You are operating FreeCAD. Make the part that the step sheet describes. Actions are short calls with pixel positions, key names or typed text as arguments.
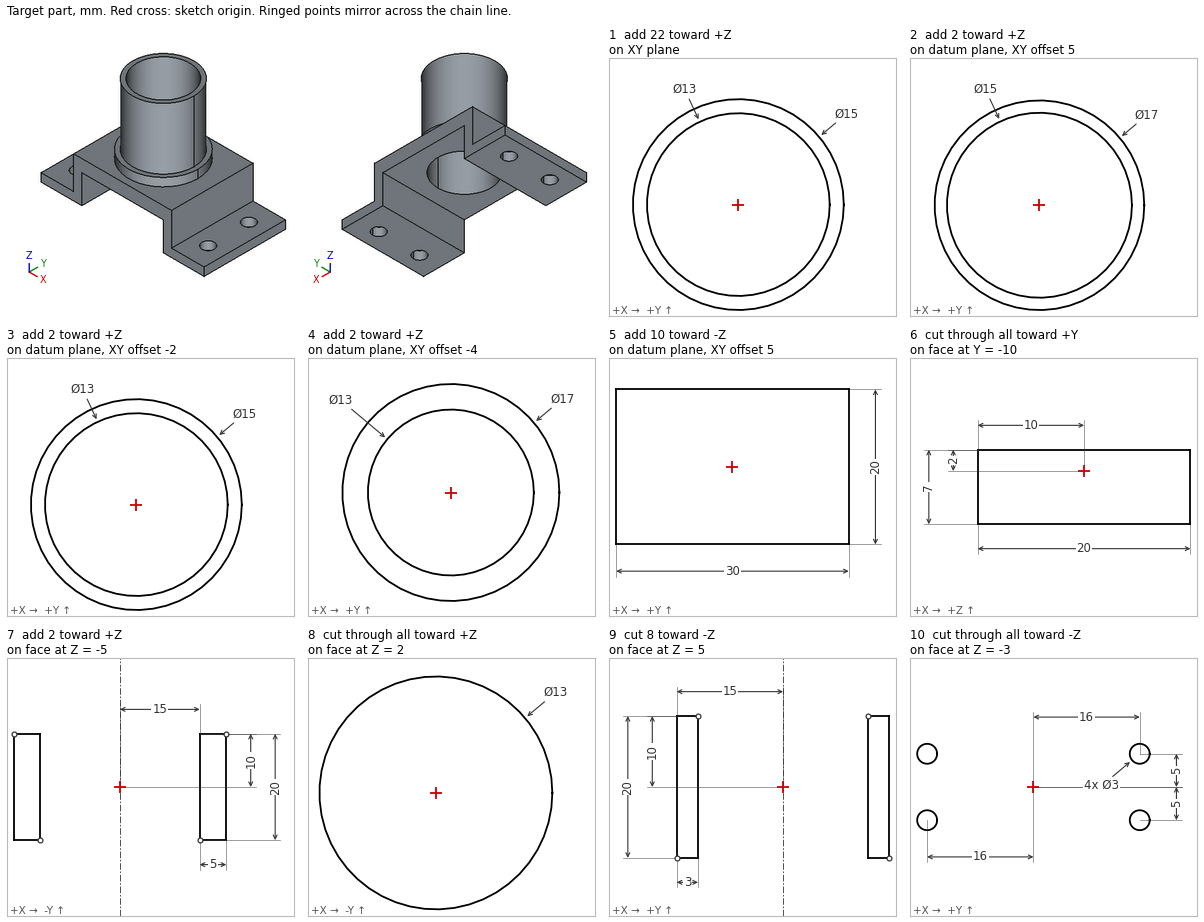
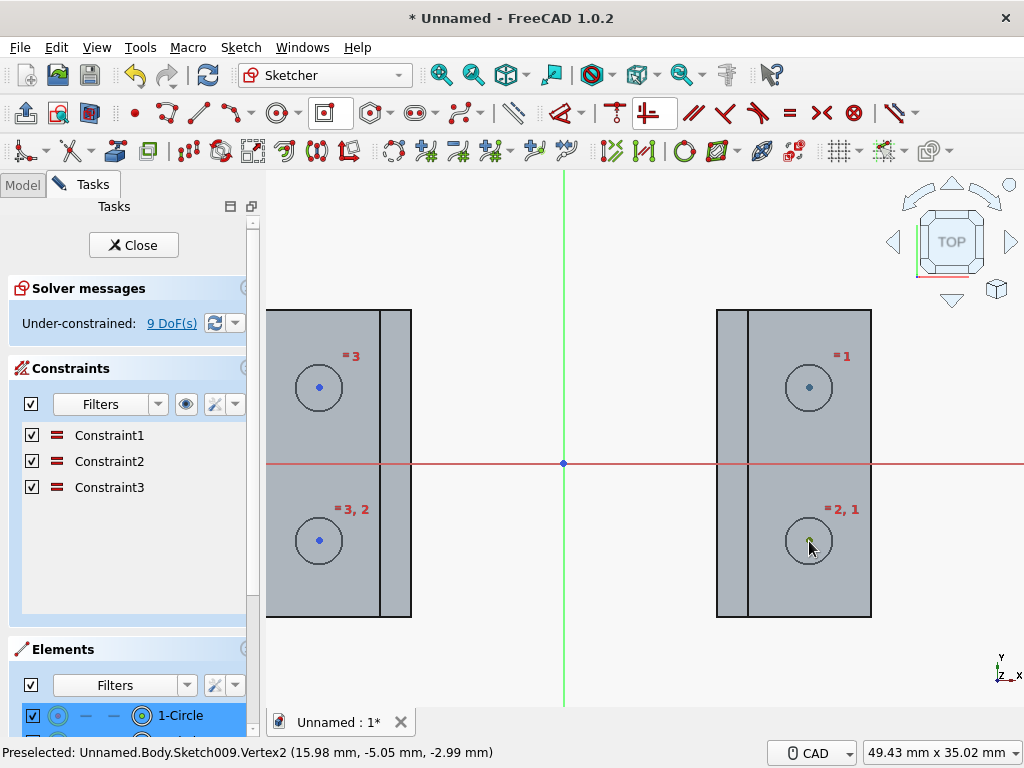
key(v)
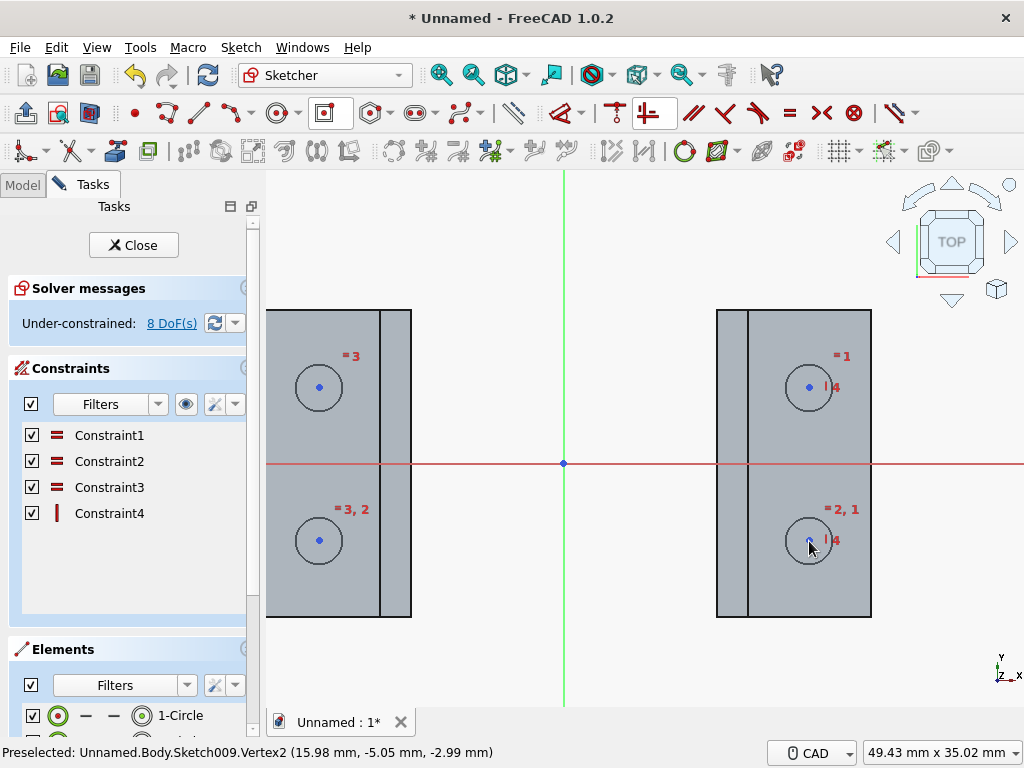
click(809, 541)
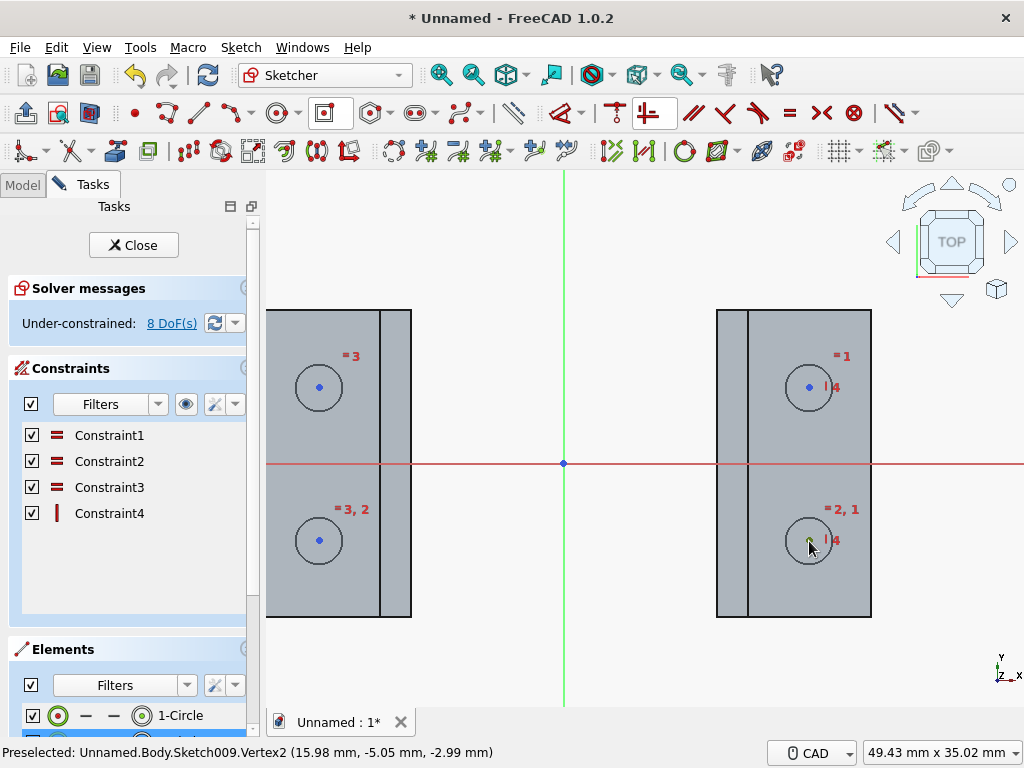
click(319, 541)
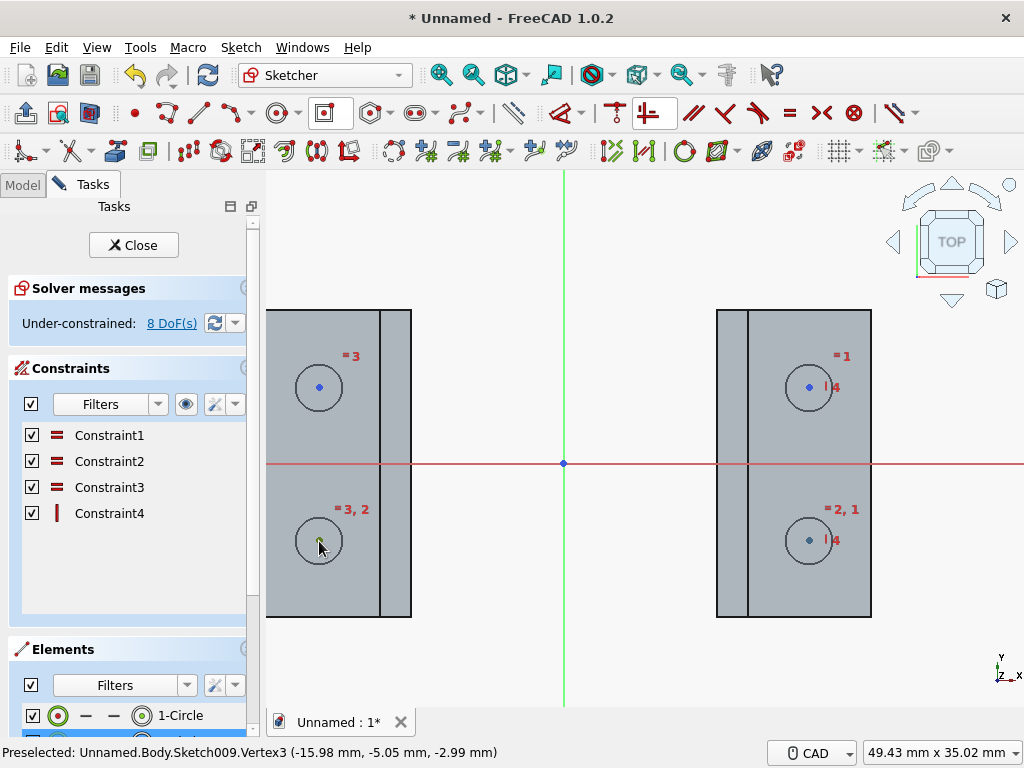
key(h)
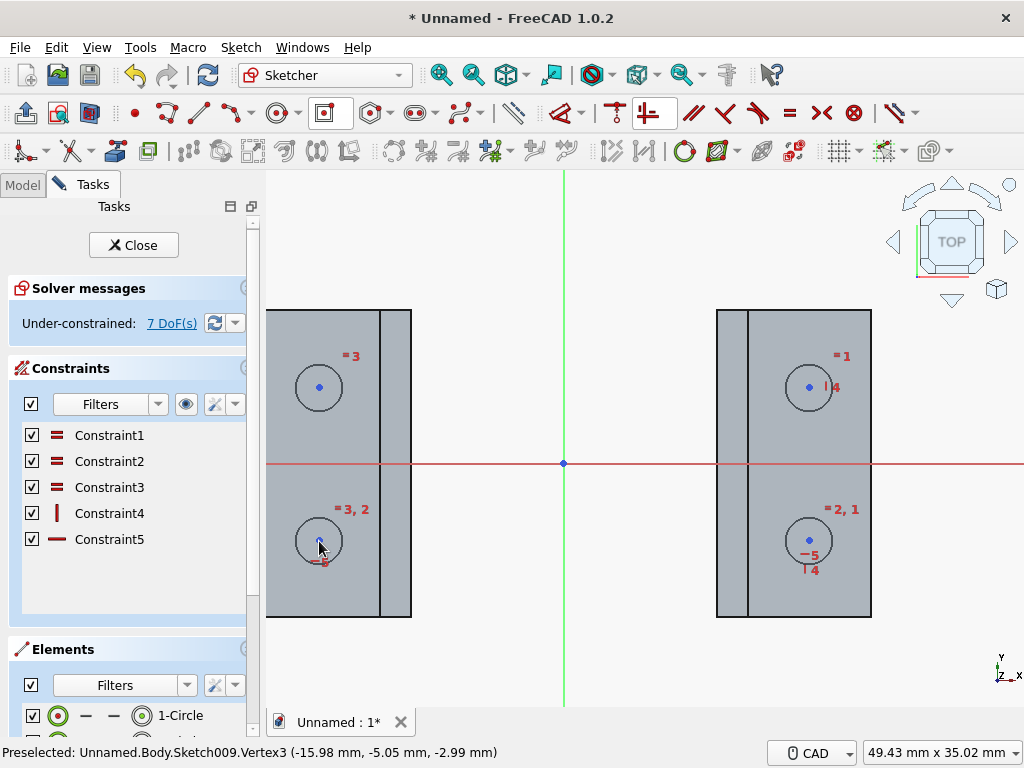
click(319, 541)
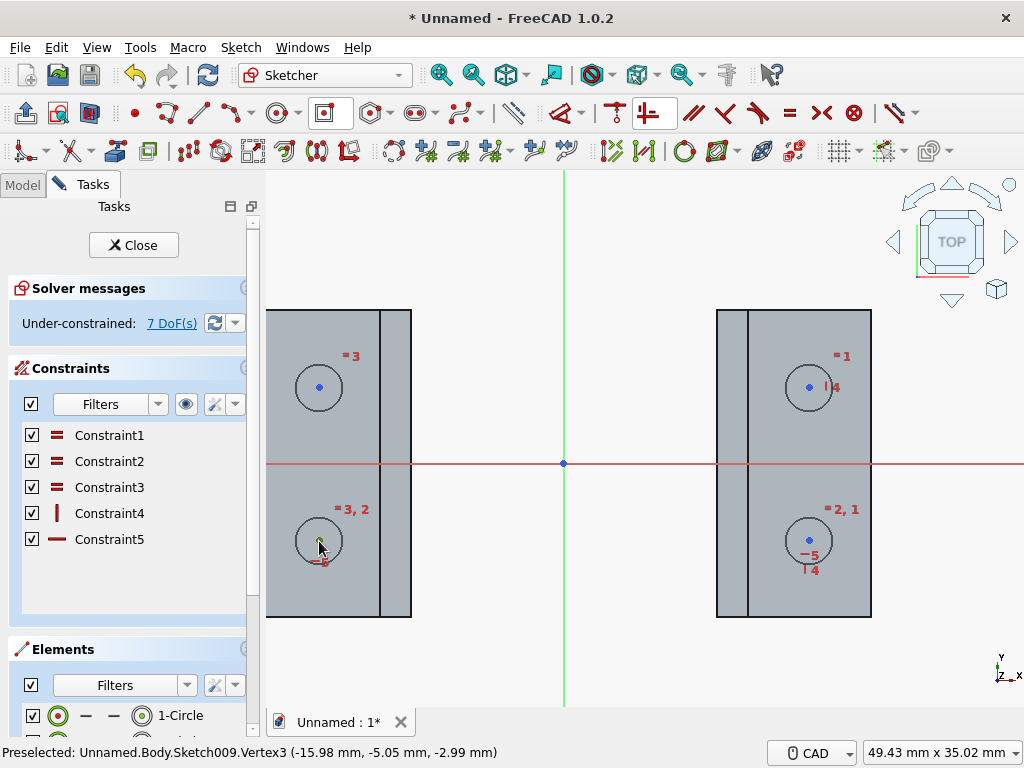
click(319, 388)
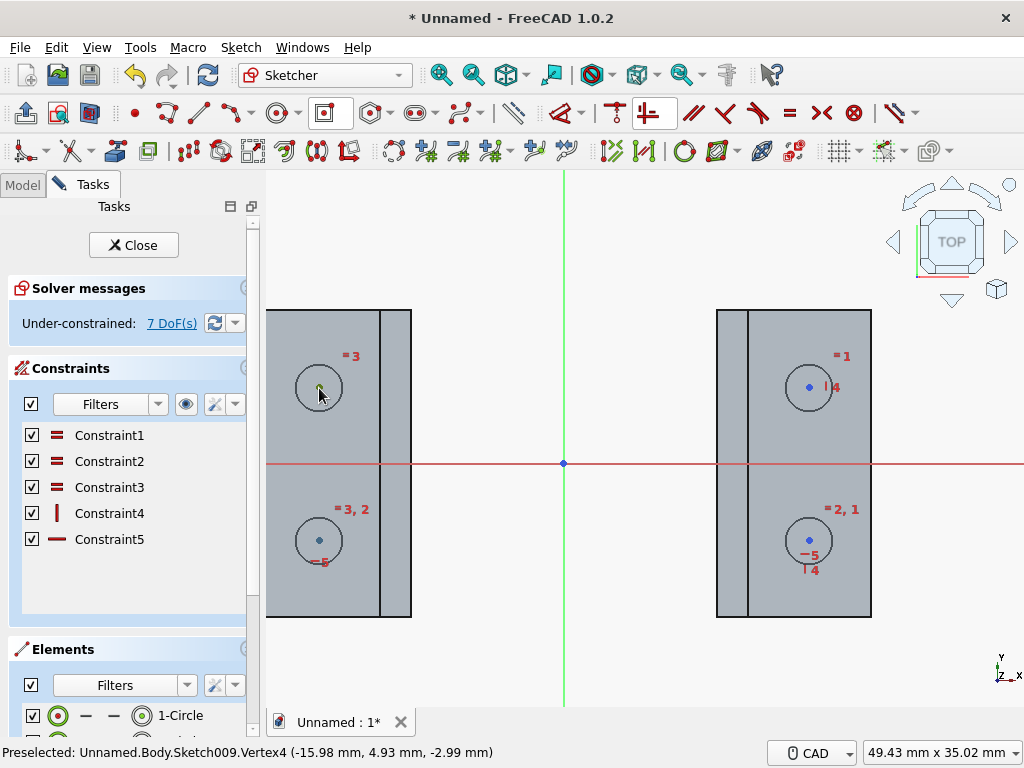
click(672, 114)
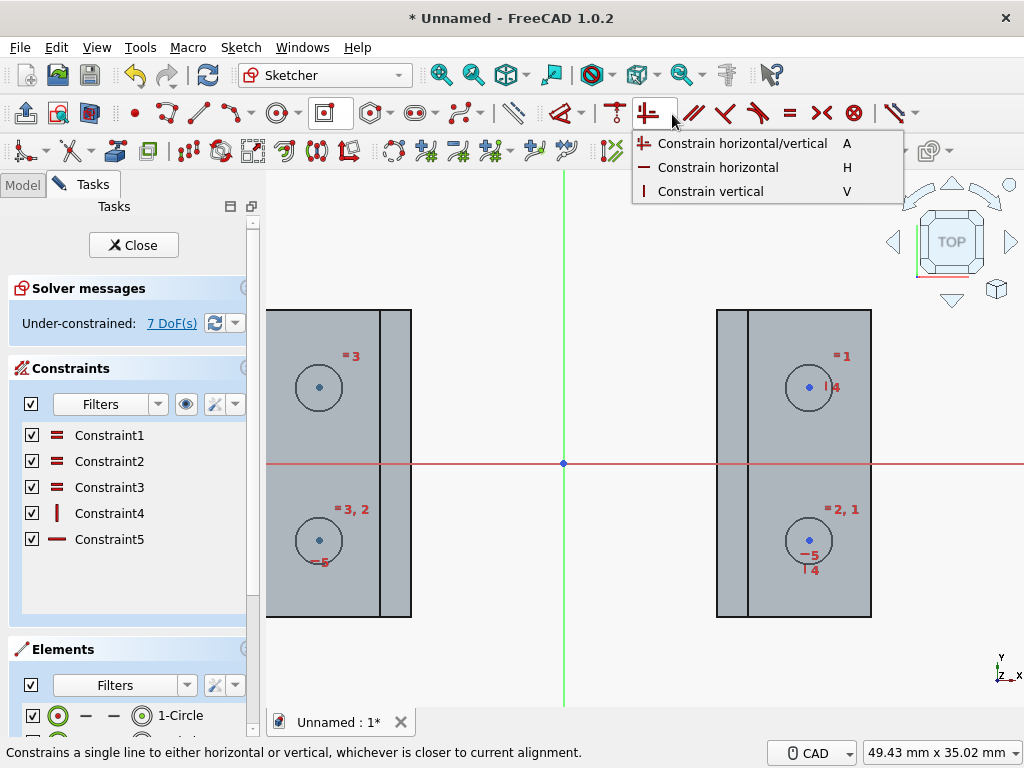
click(768, 191)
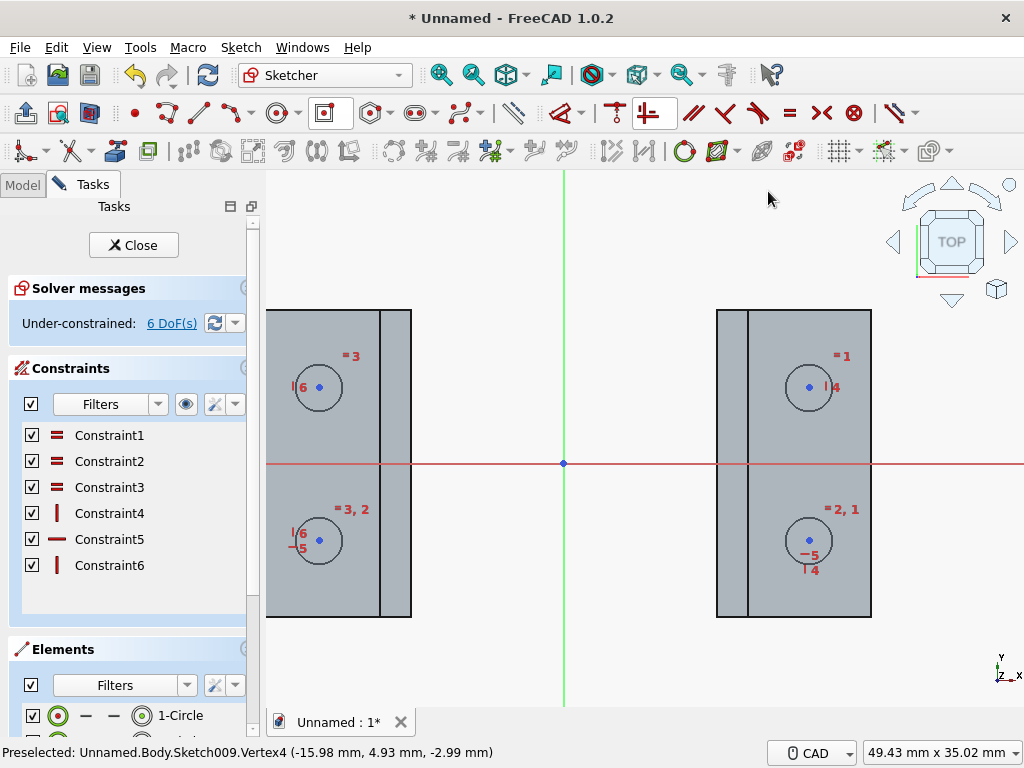
click(809, 388)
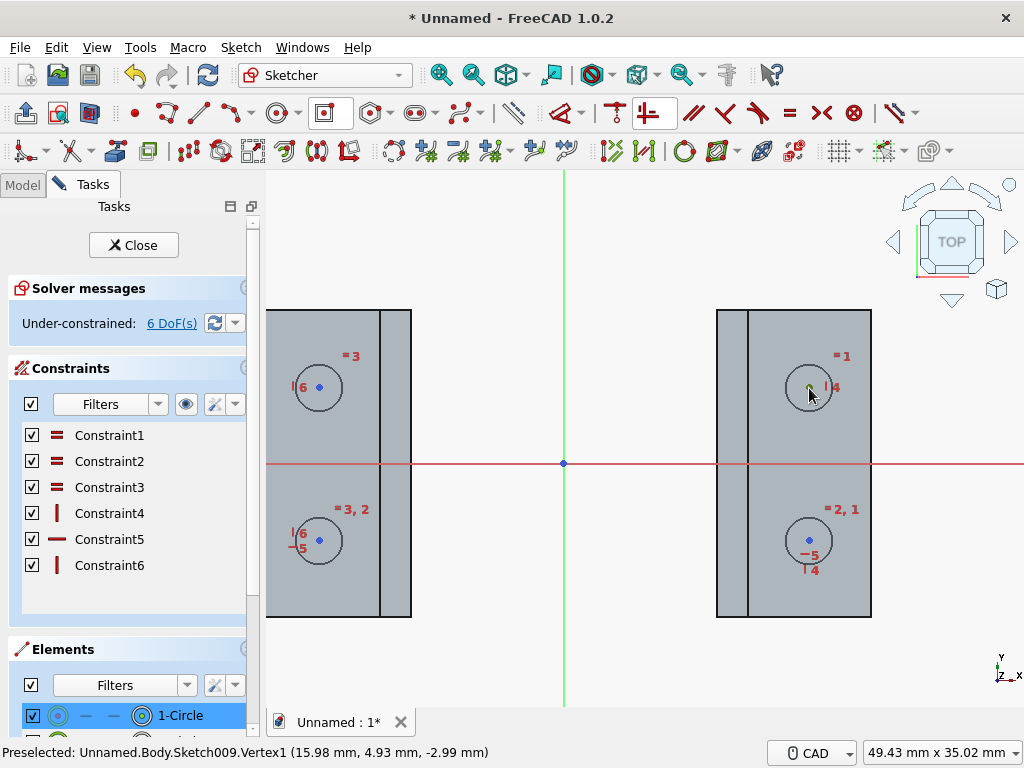
click(319, 388)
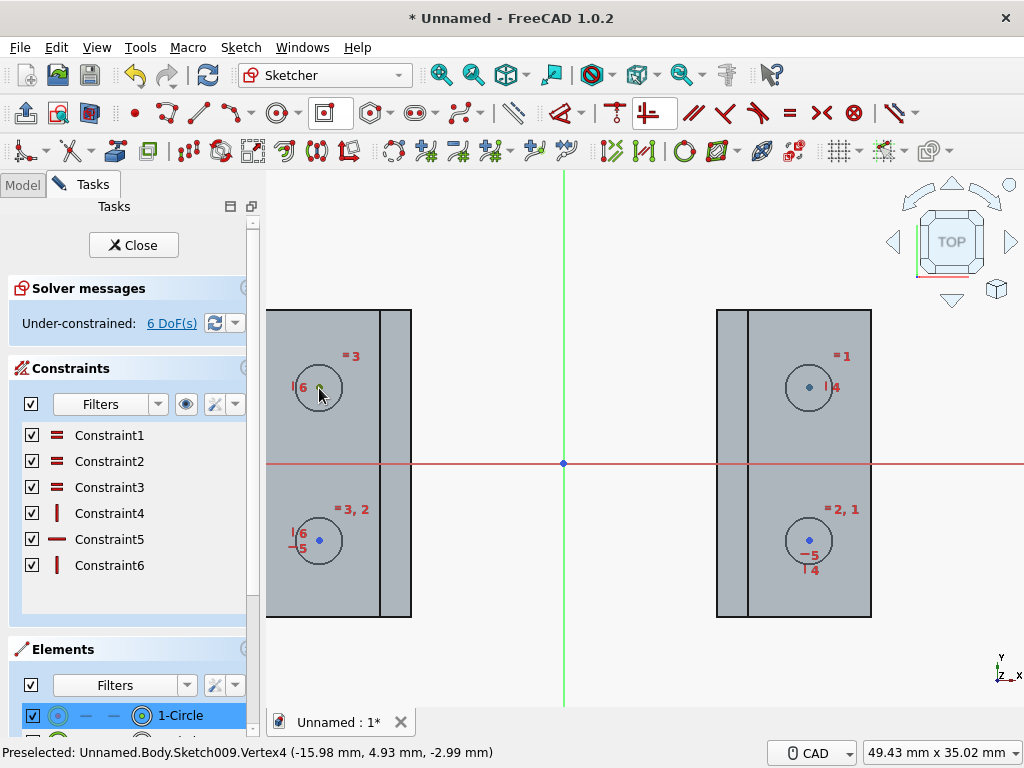
click(672, 114)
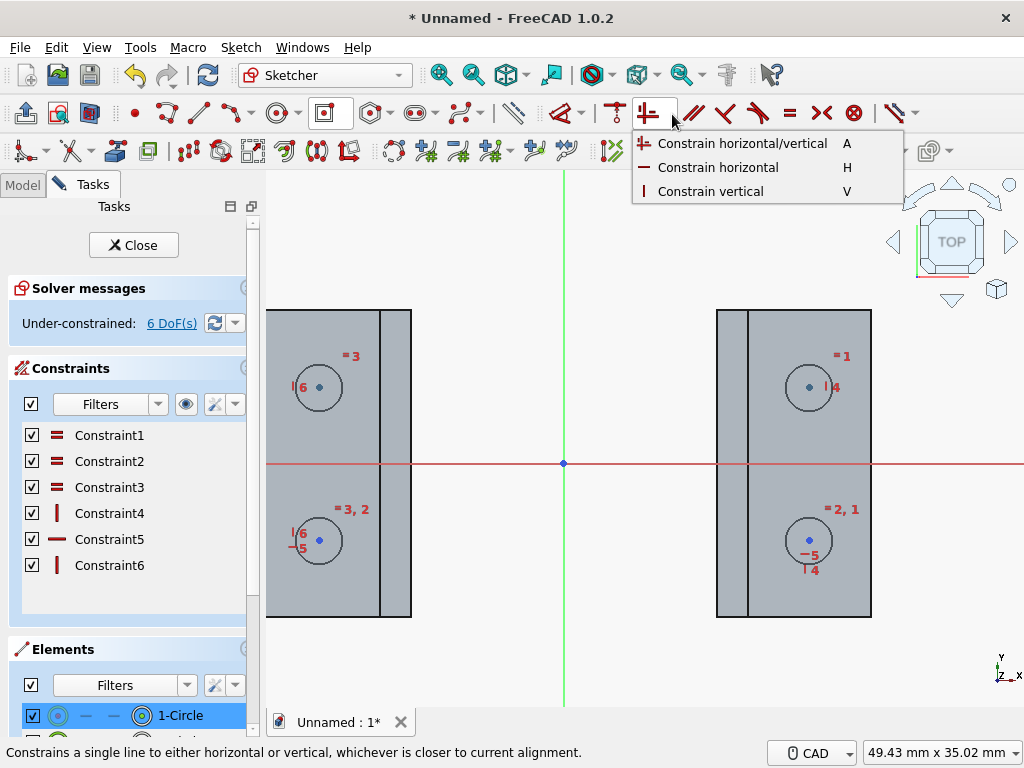
click(768, 167)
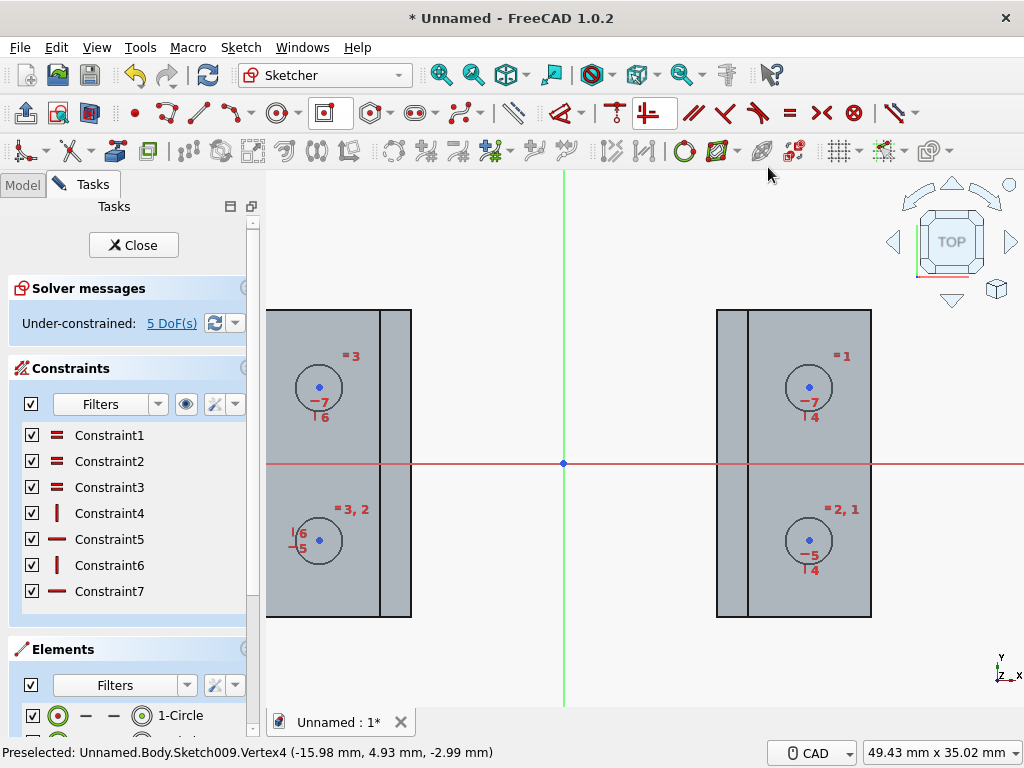
key(d)